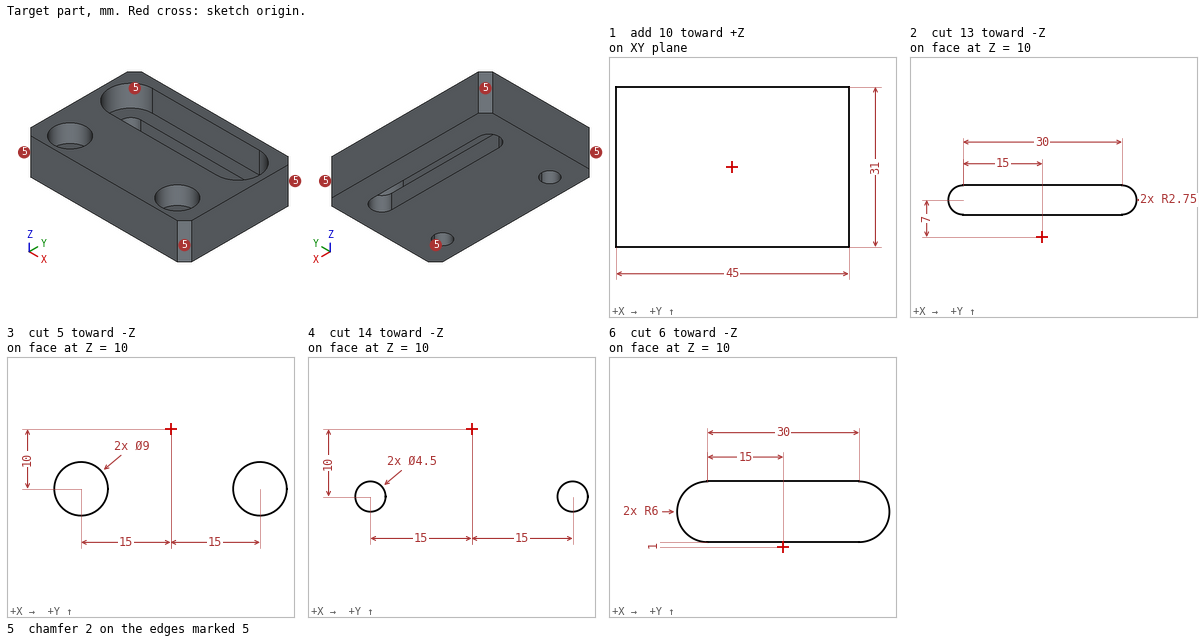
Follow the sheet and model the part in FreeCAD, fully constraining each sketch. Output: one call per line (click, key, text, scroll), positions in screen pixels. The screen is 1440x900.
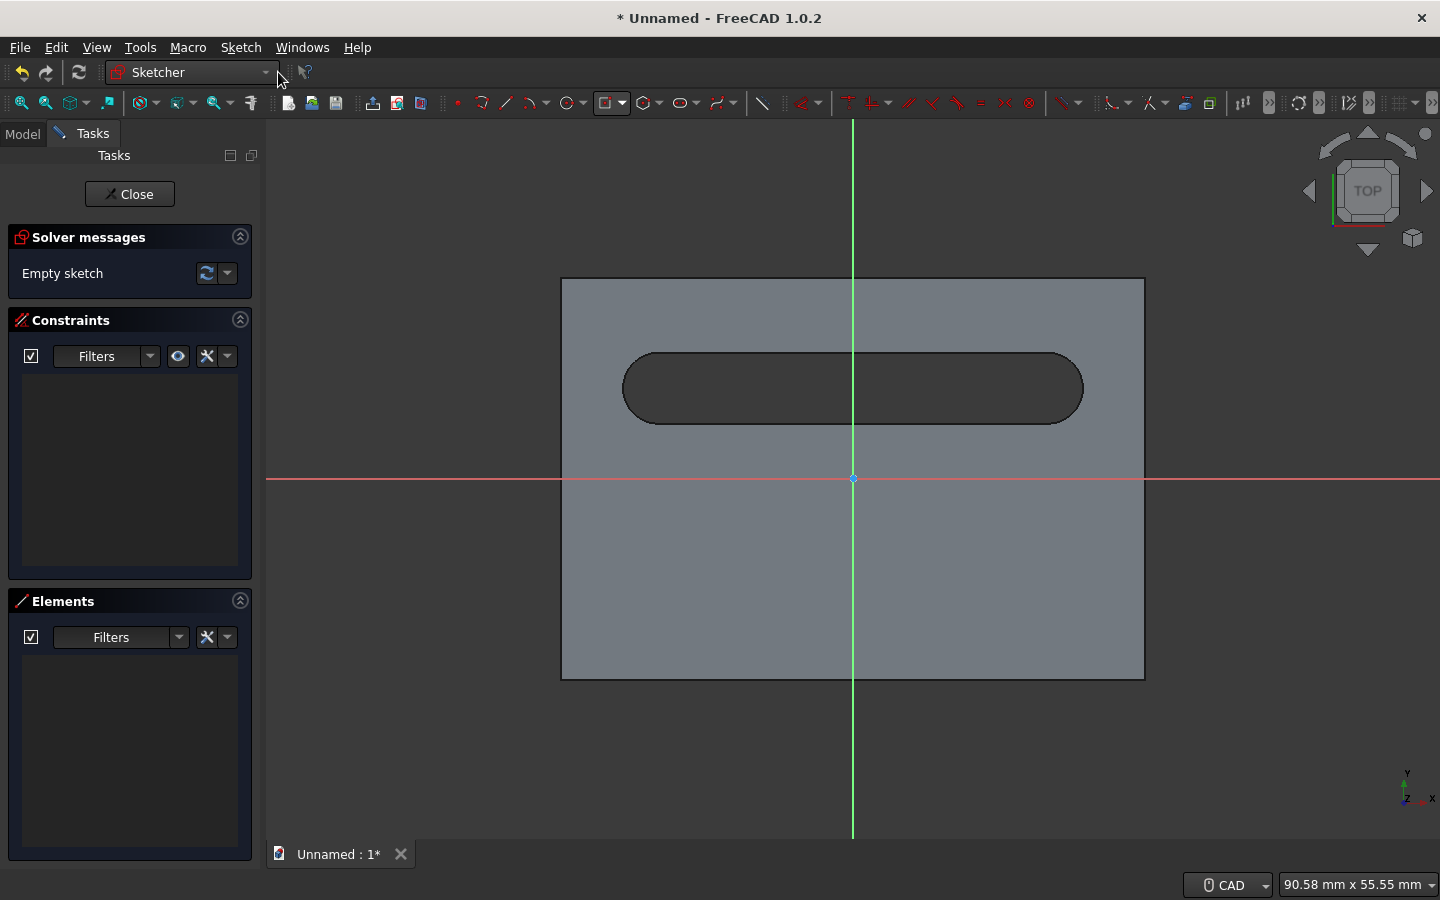
scroll(992, 764, up, 2)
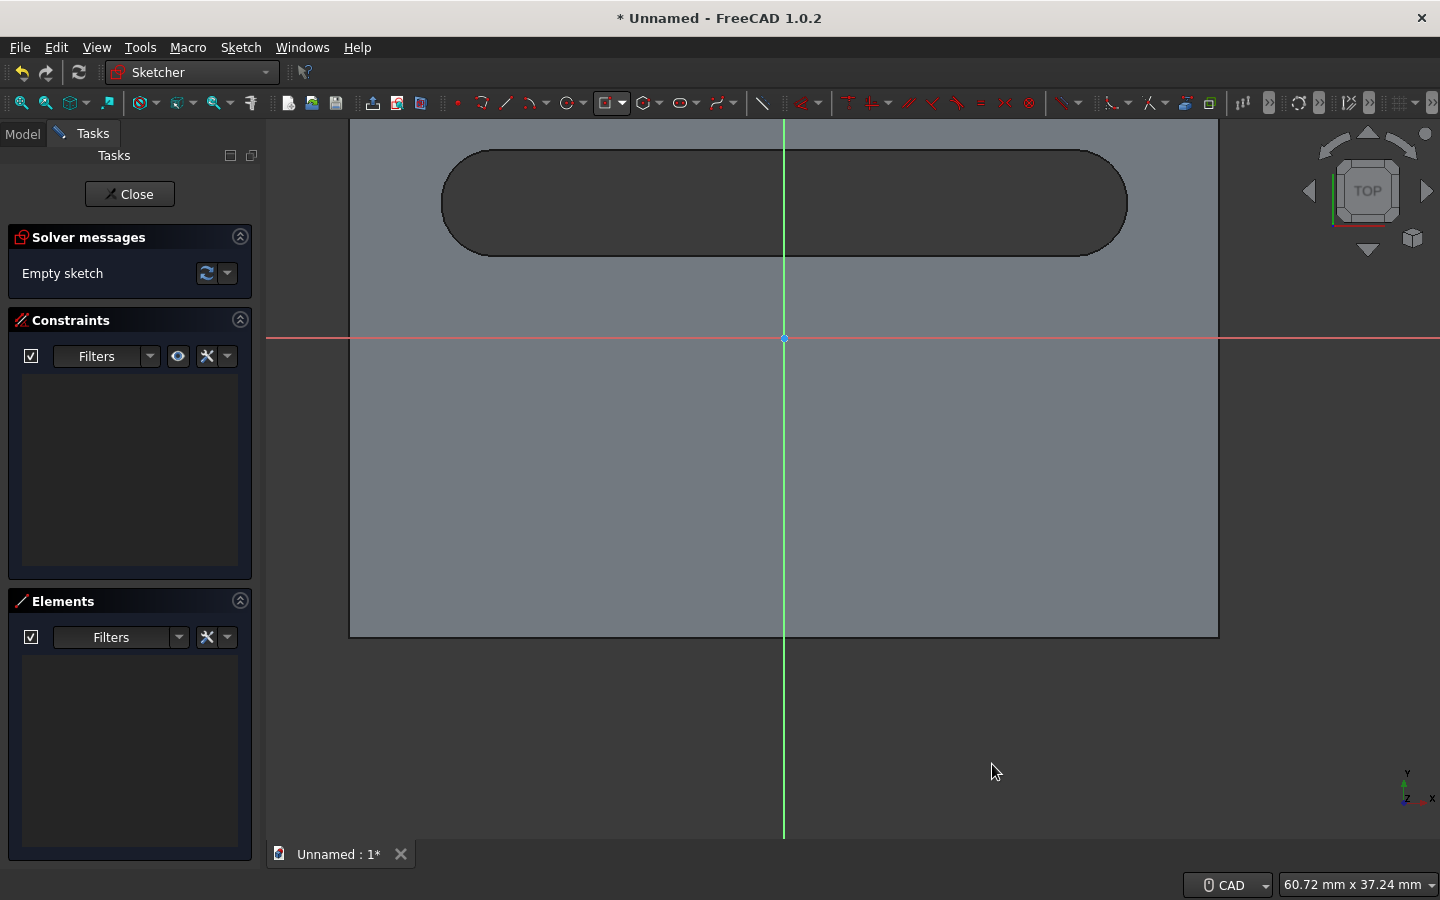
click(568, 104)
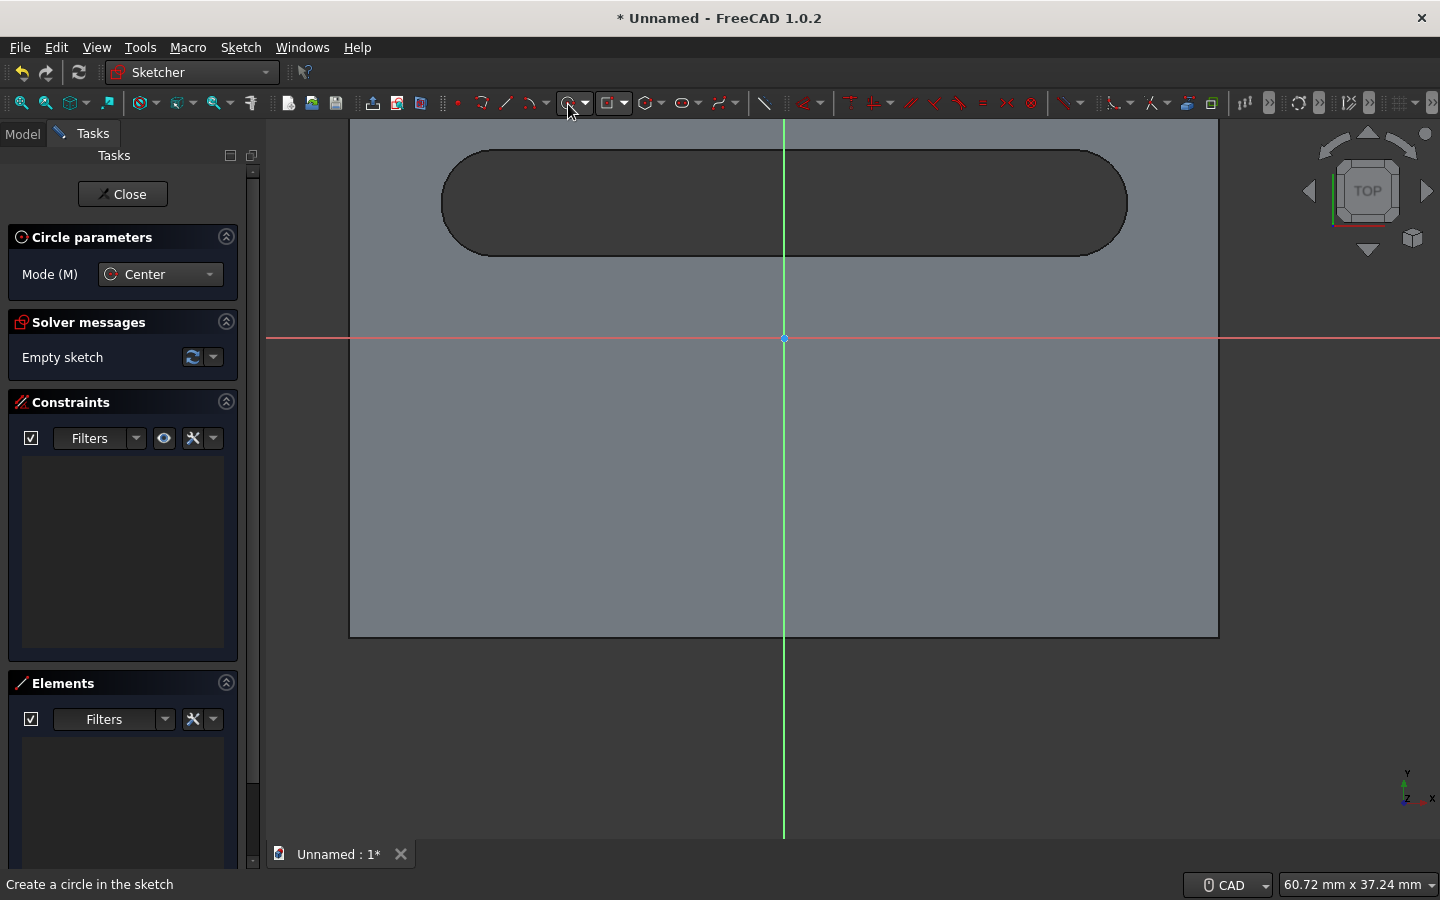
click(494, 532)
click(556, 470)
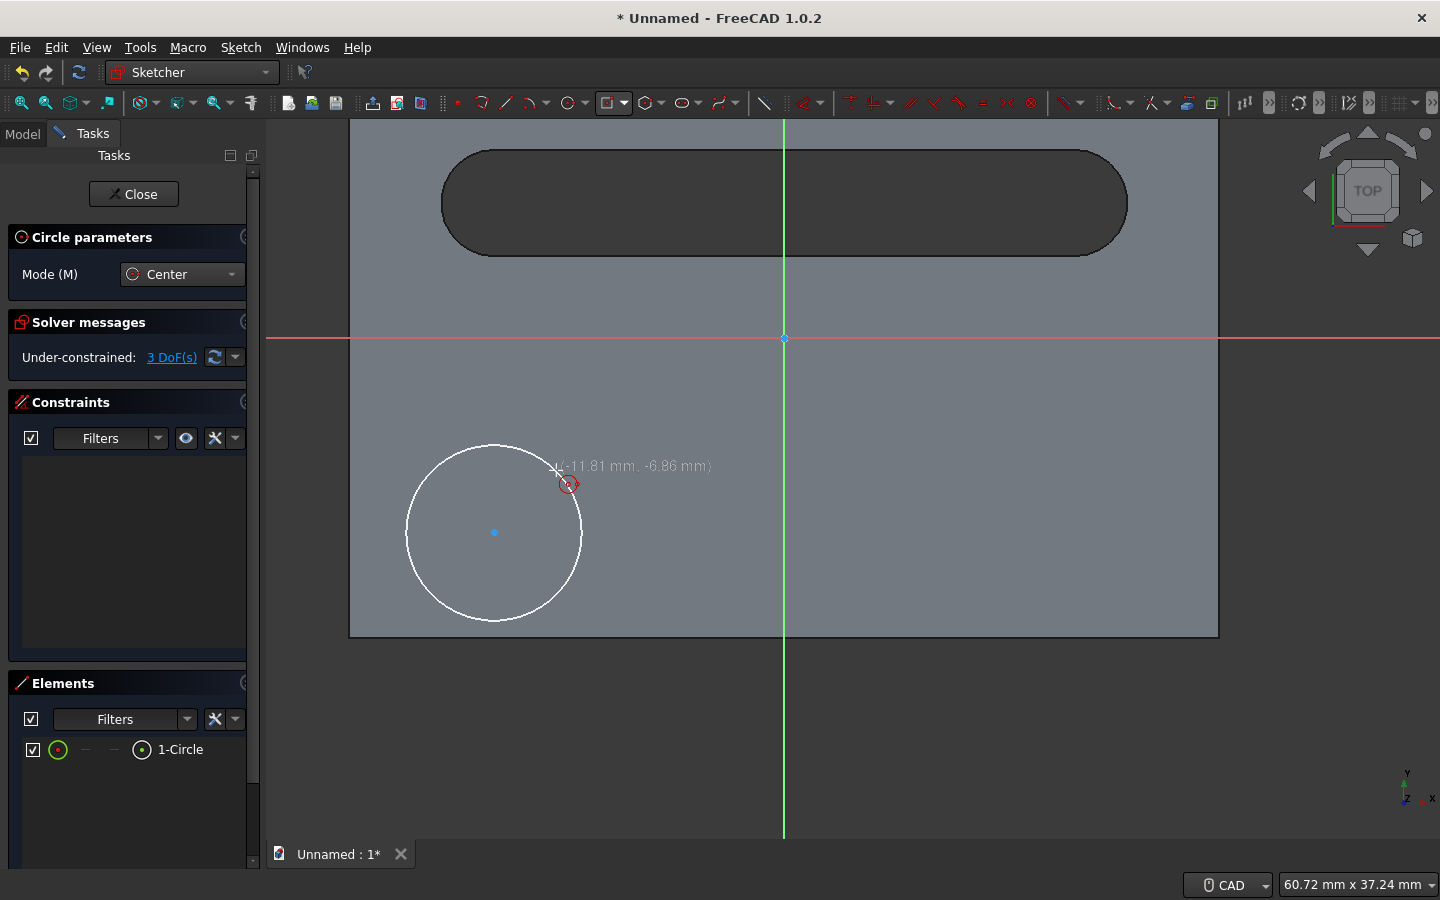
click(1074, 532)
click(1136, 470)
key(Escape)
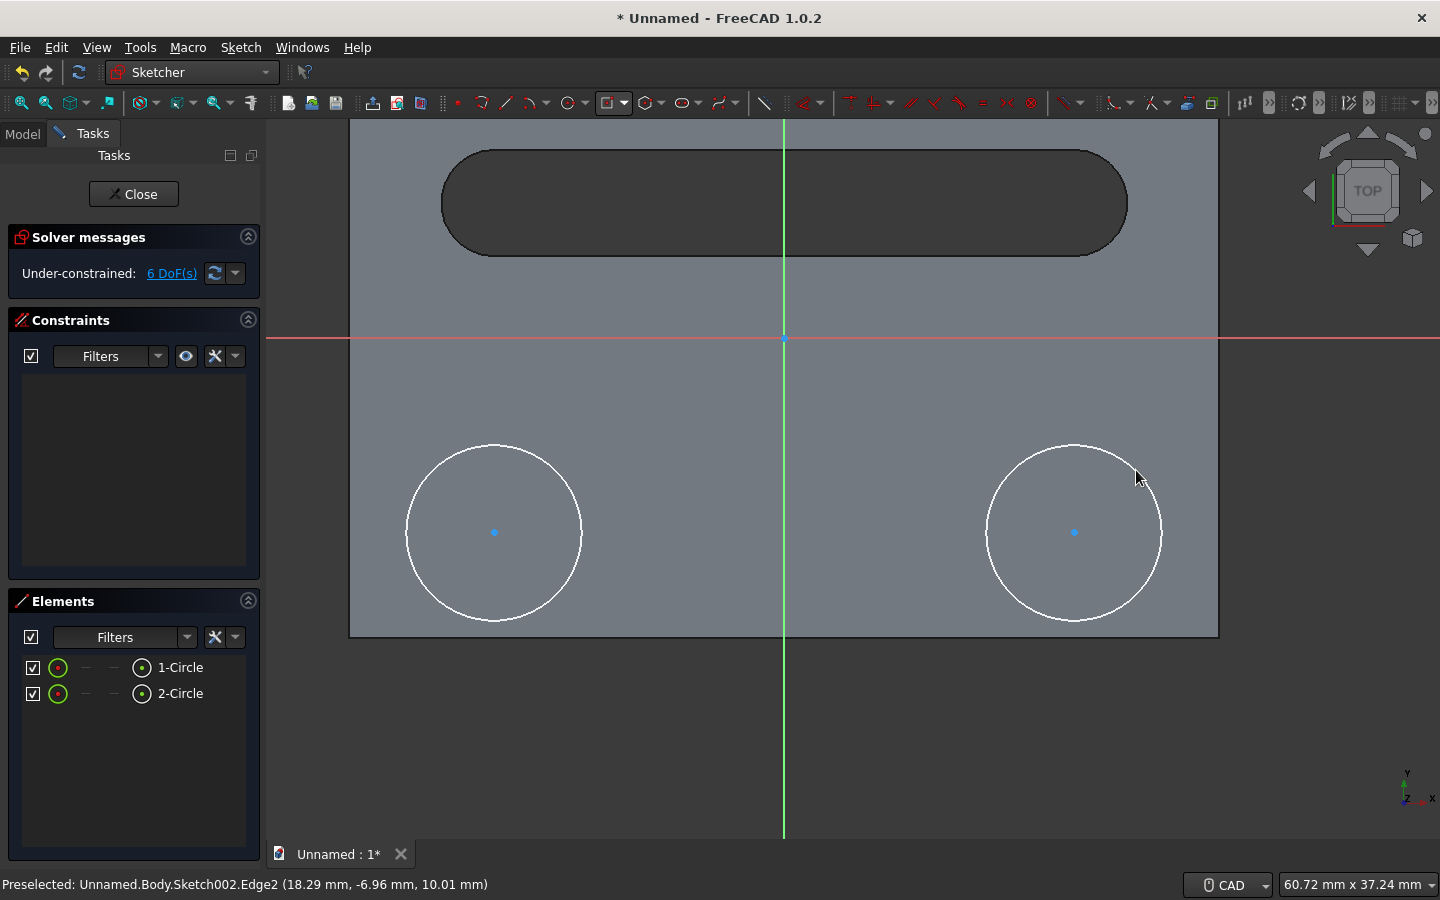
click(556, 471)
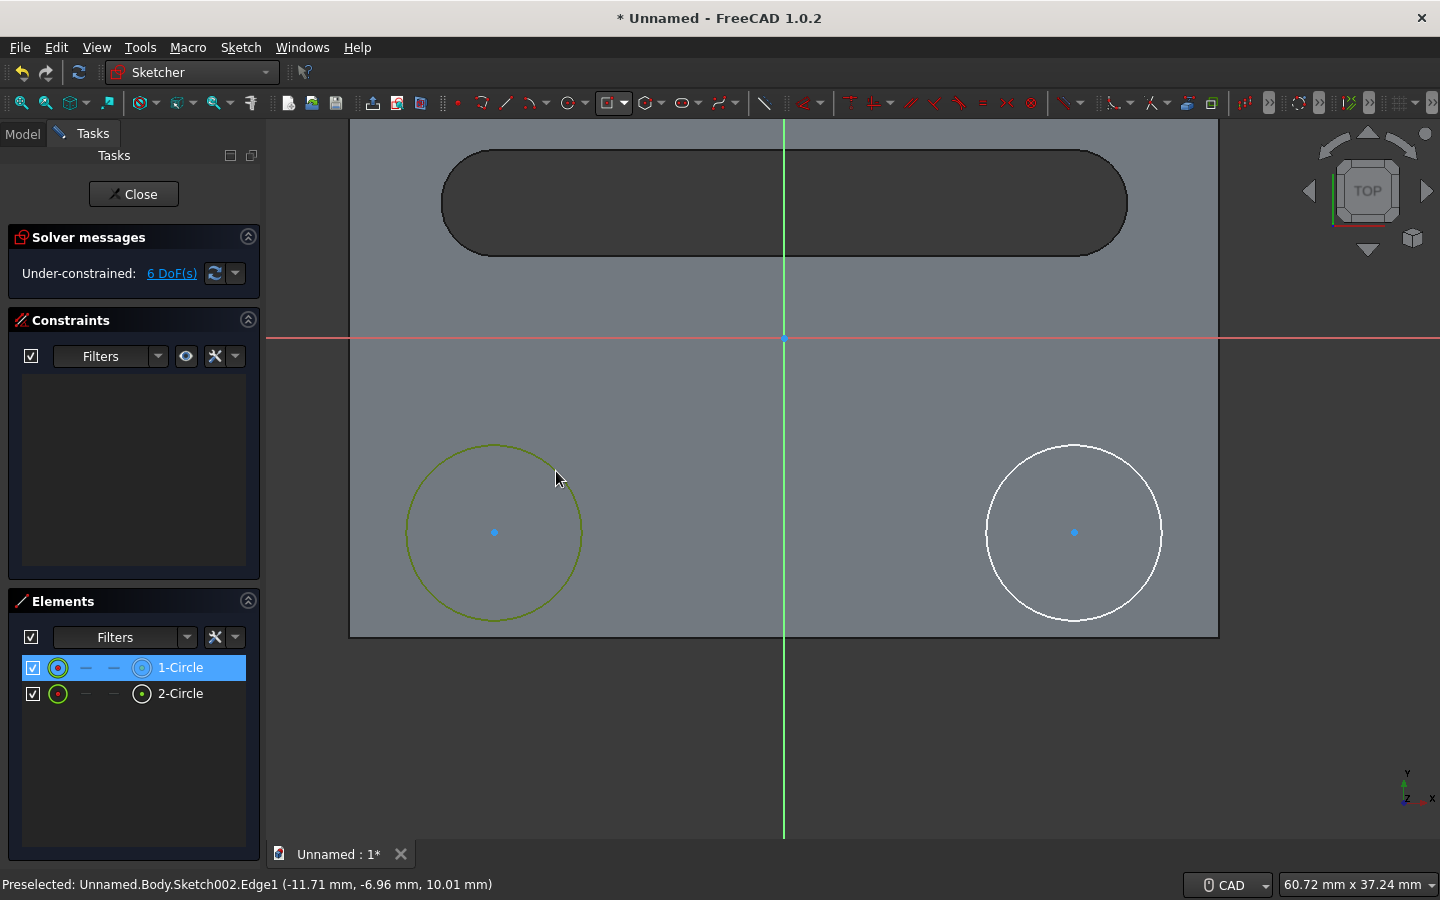
click(1136, 471)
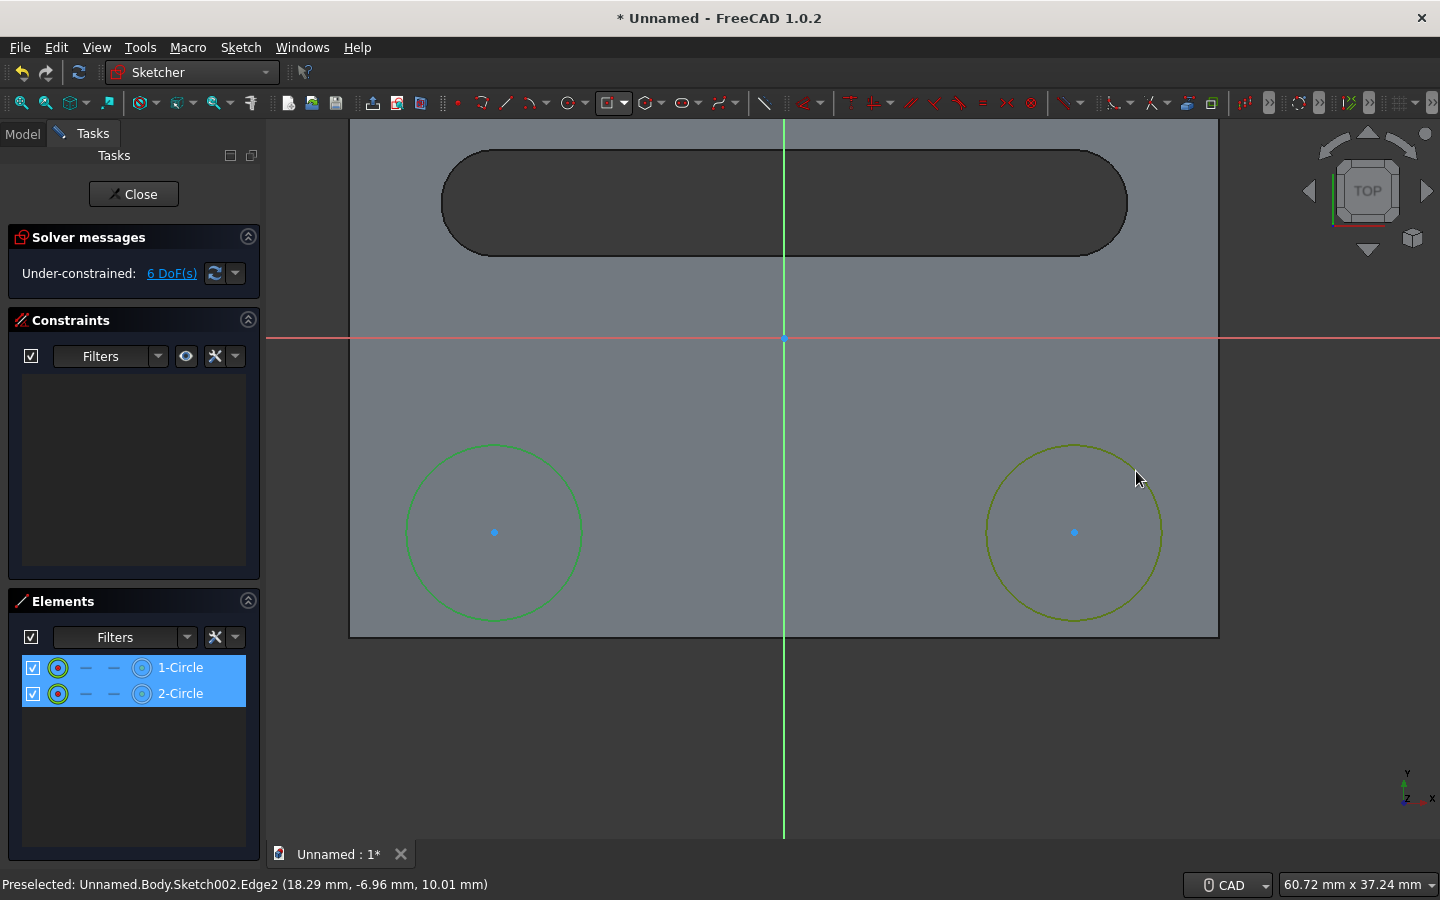
click(984, 104)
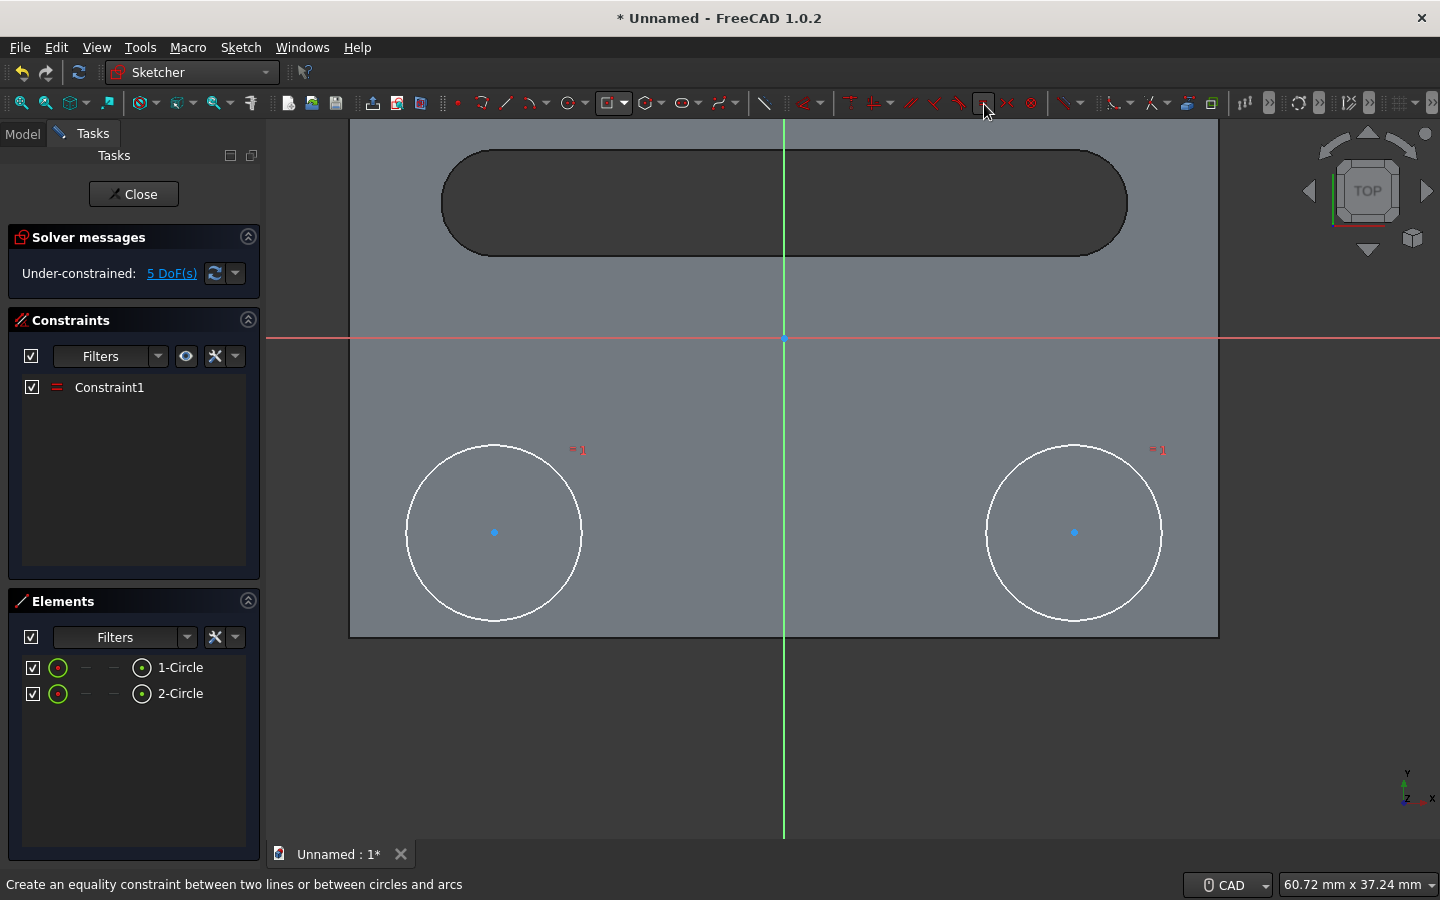
click(494, 533)